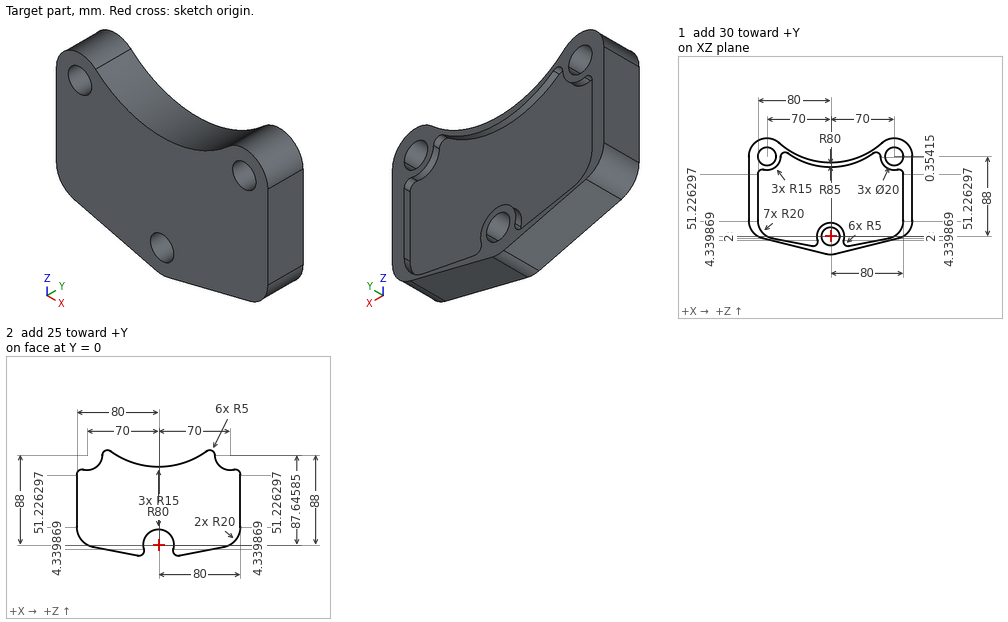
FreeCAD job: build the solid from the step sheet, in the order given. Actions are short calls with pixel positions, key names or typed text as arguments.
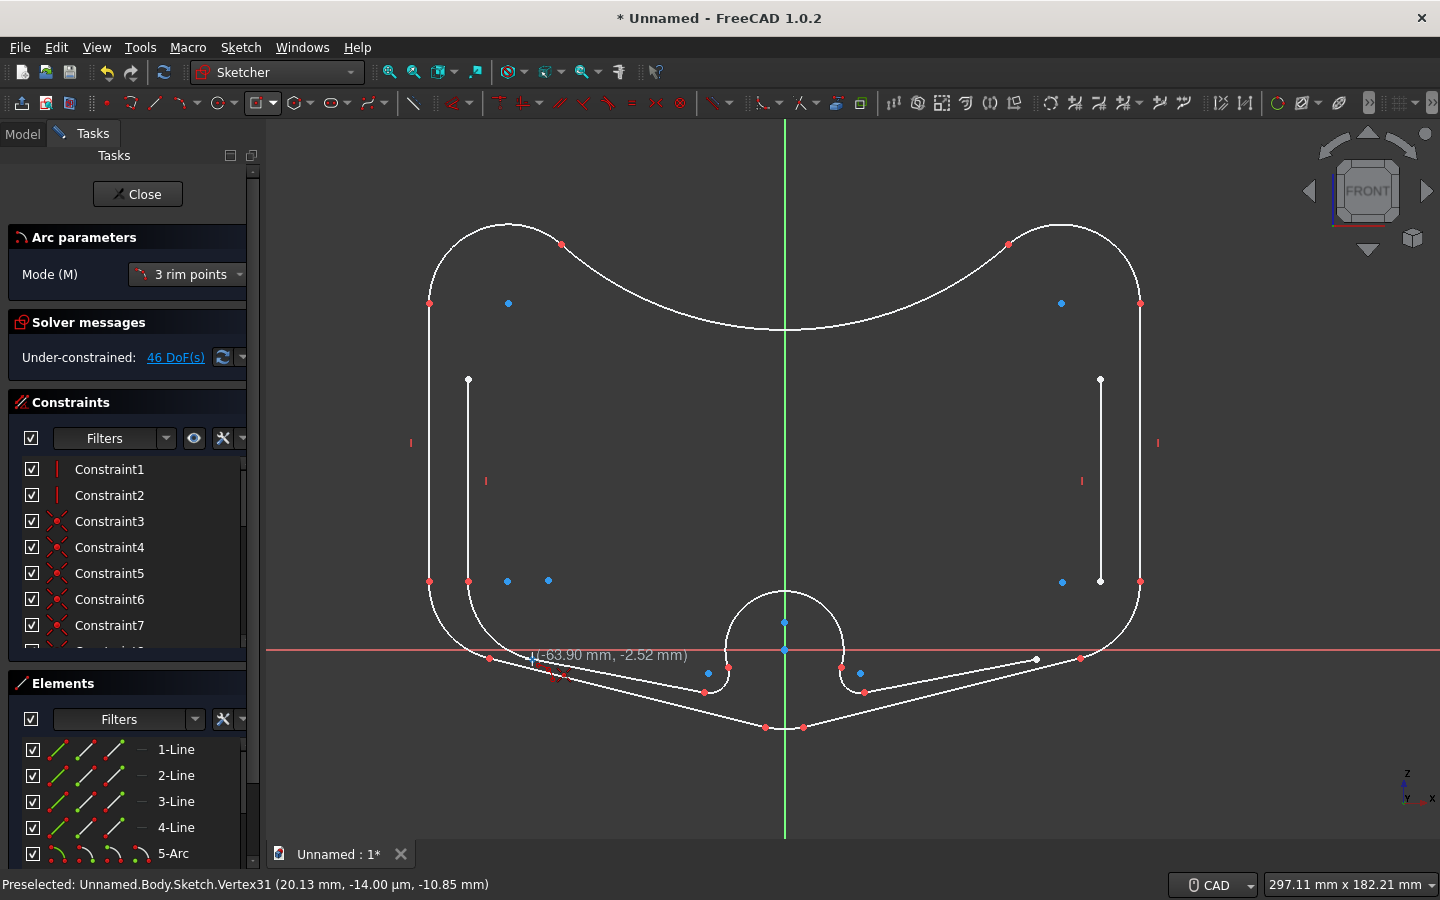
scroll(1037, 659, up, 3)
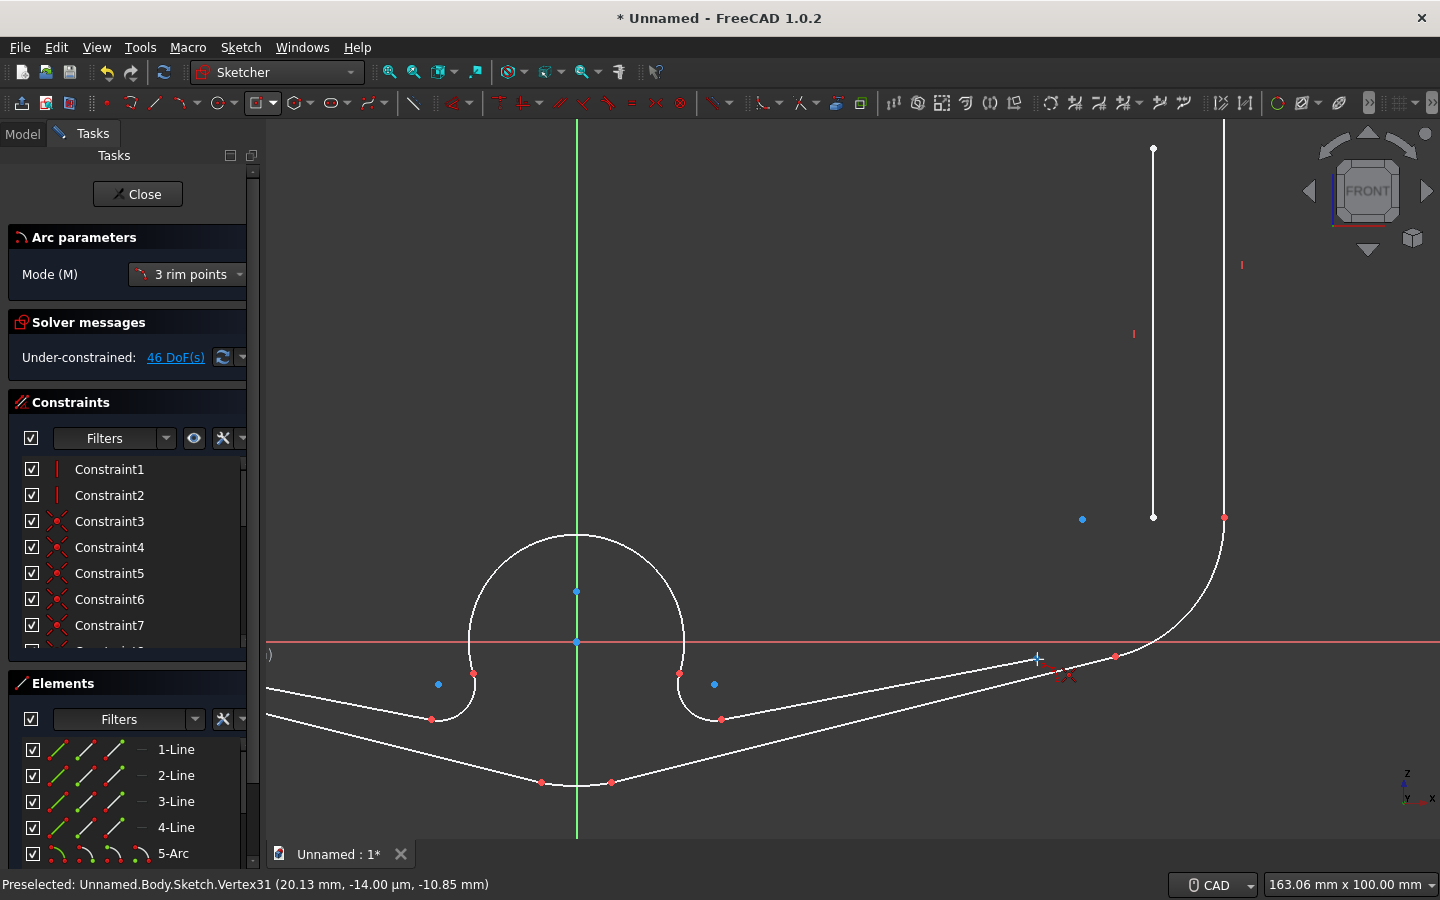
click(1036, 659)
click(1153, 518)
click(1120, 608)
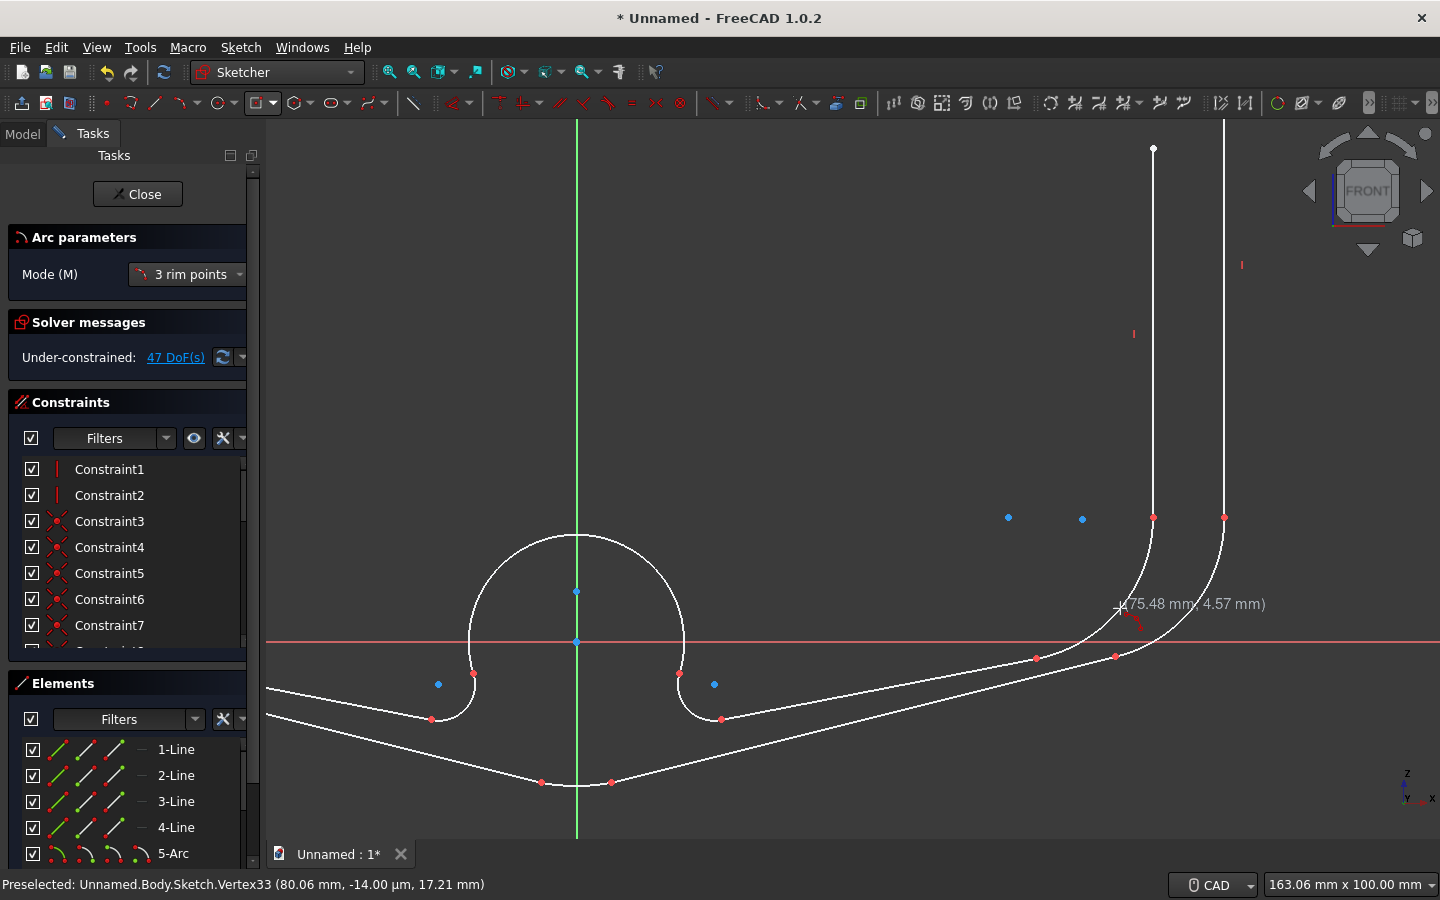
click(1153, 149)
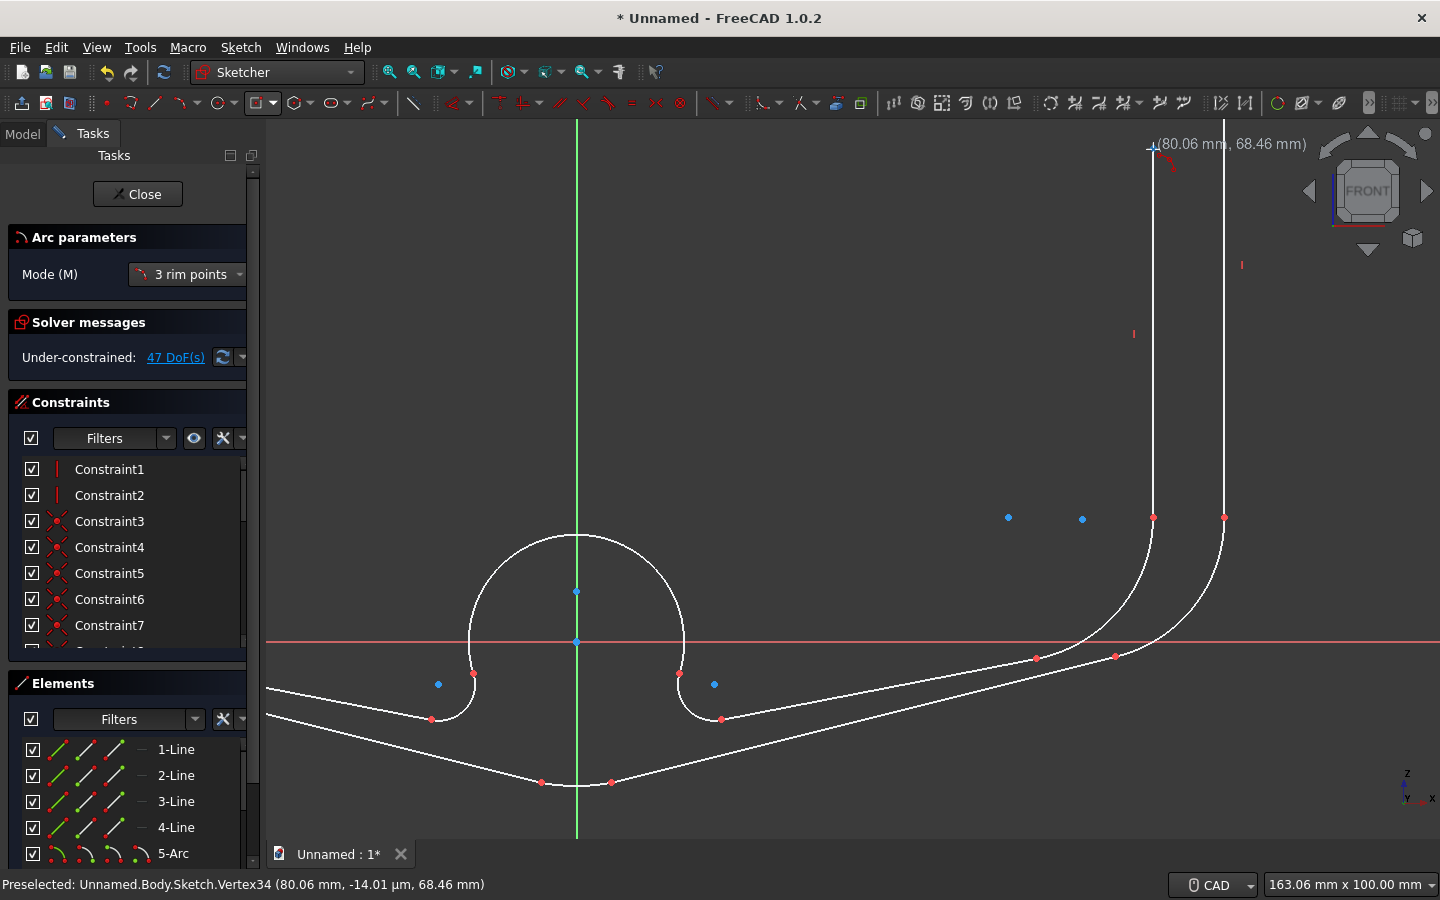
scroll(1037, 659, down, 3)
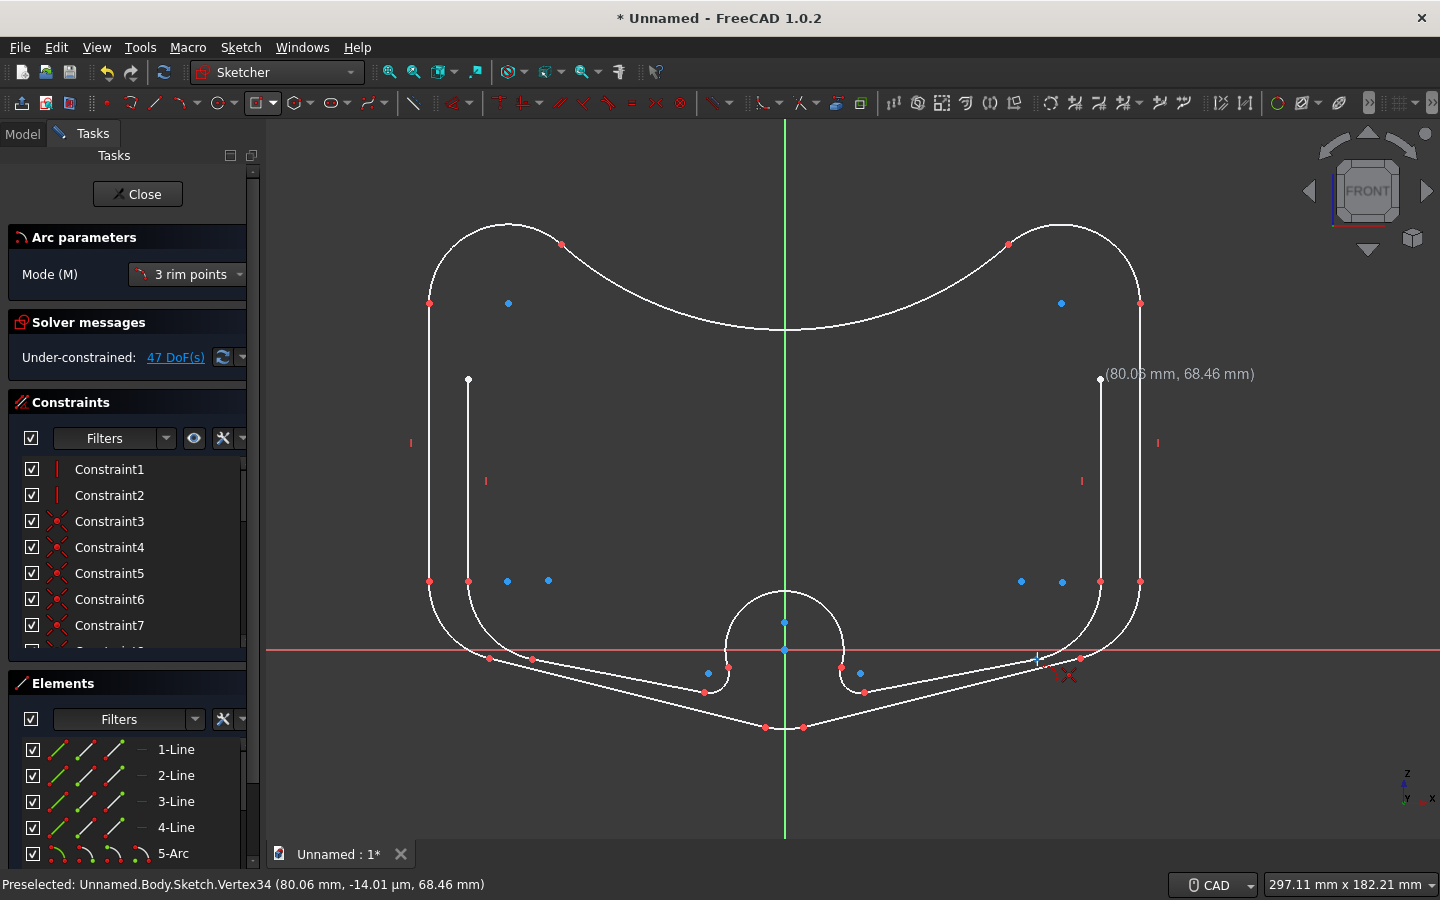
click(1076, 360)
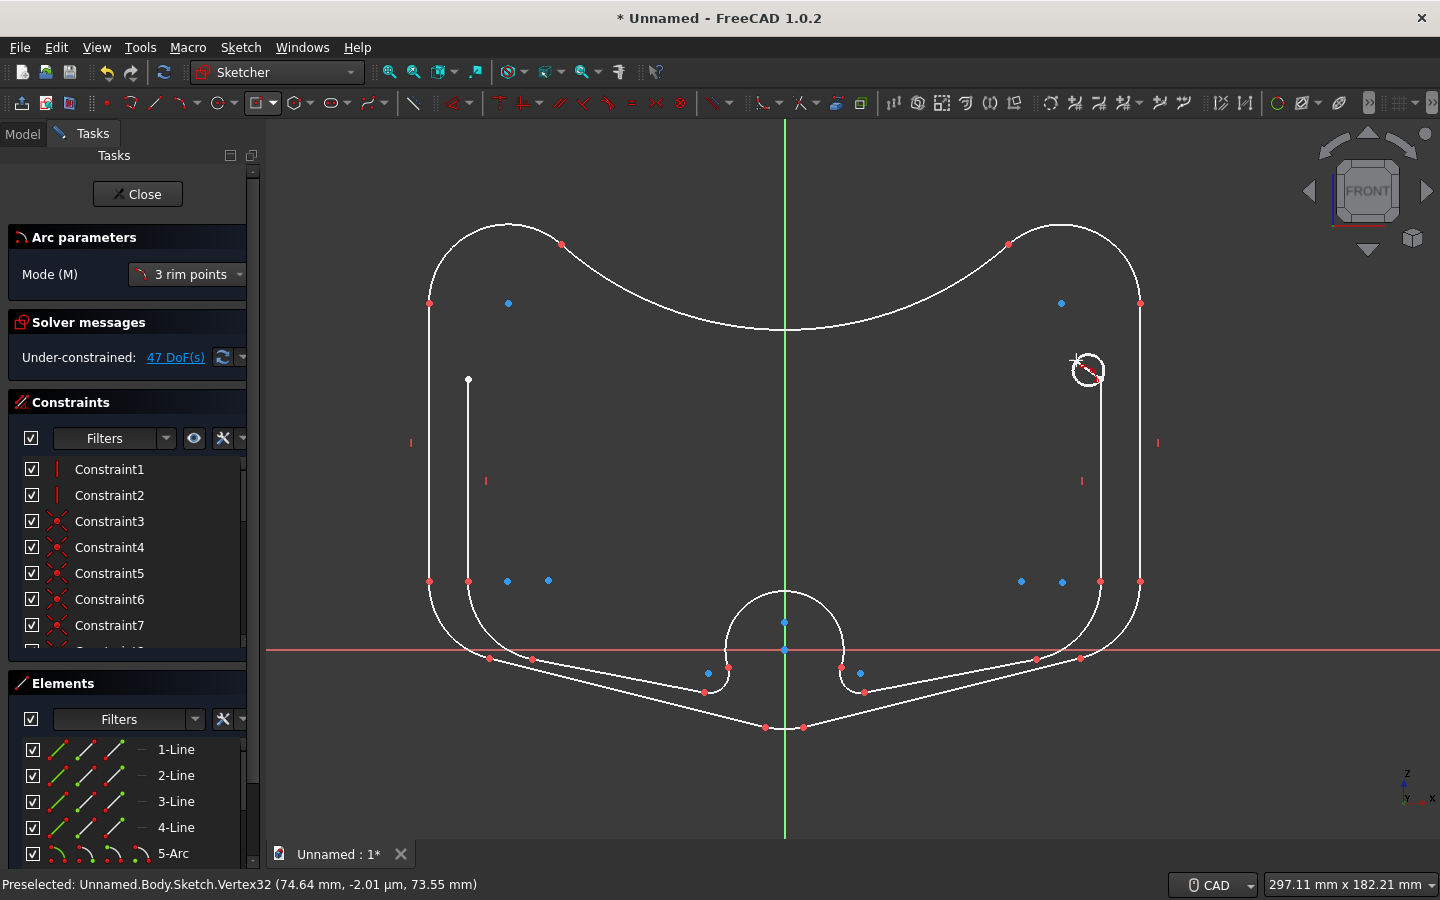
scroll(1093, 363, up, 4)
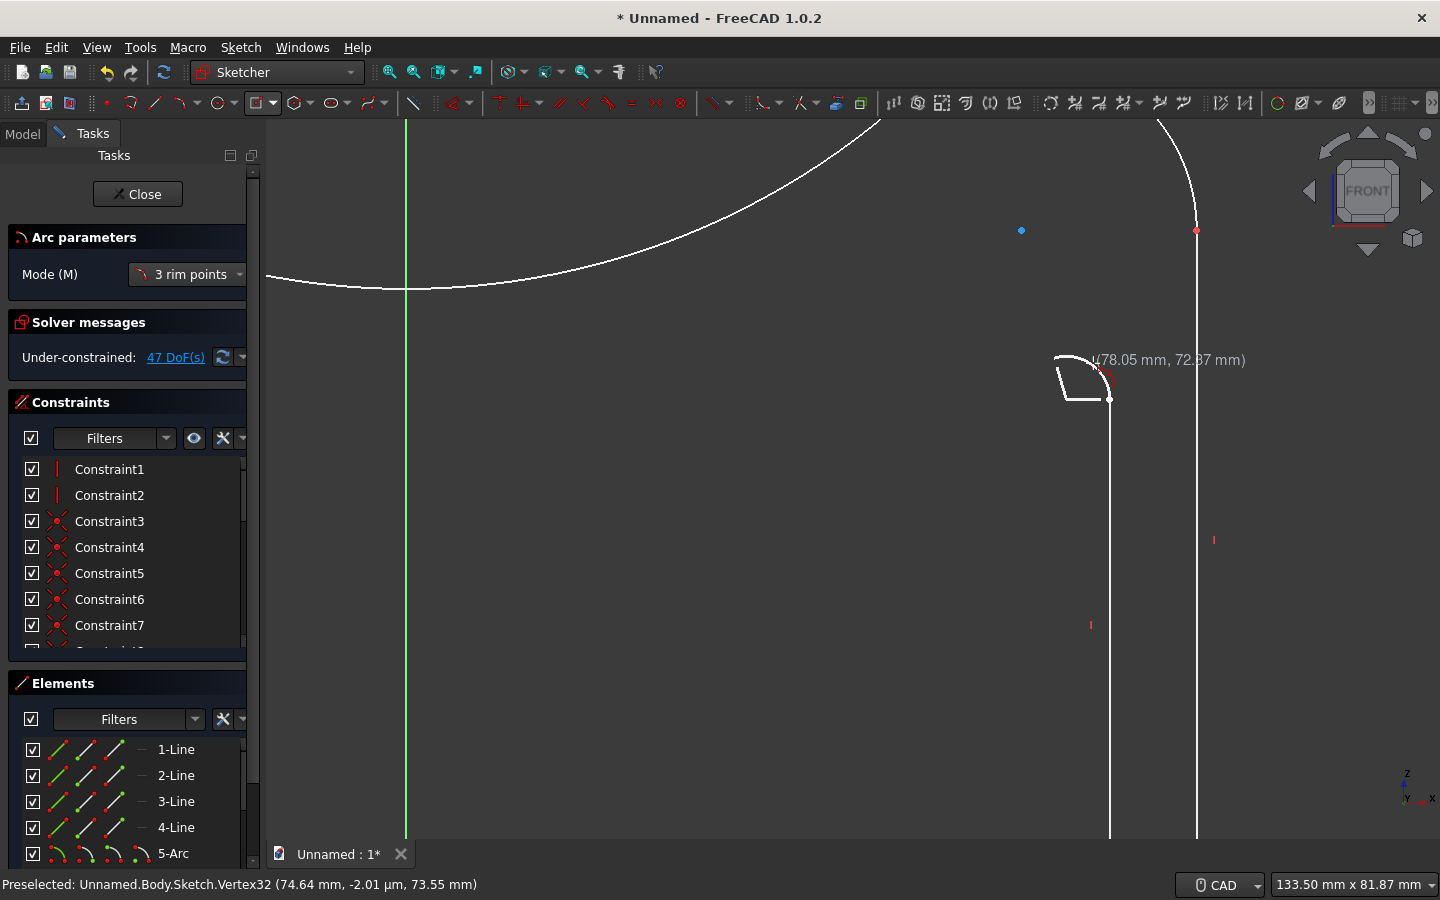
click(1092, 363)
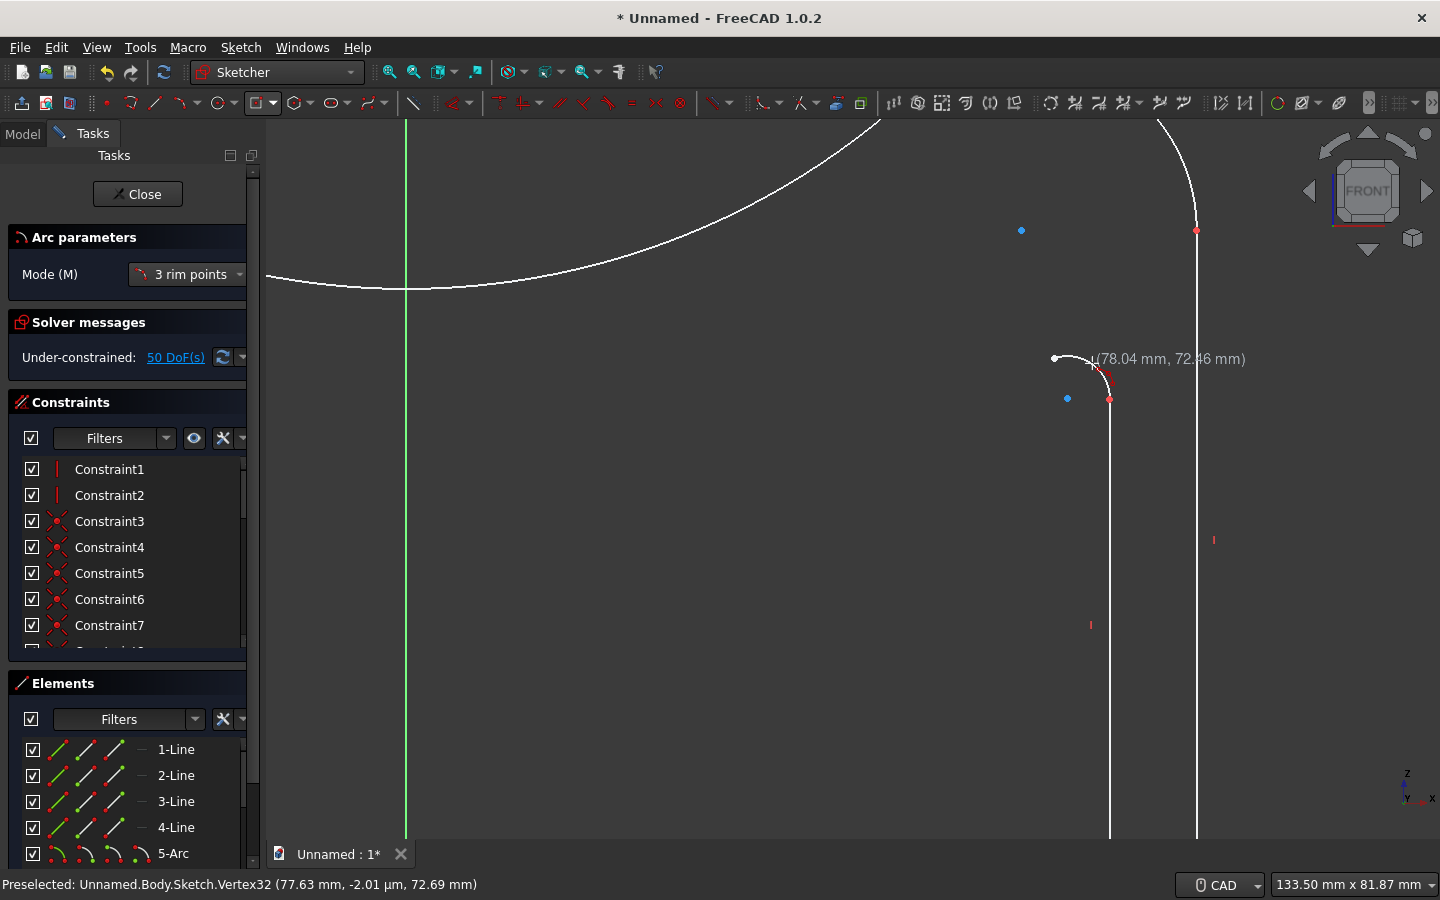
click(1054, 358)
click(889, 230)
click(942, 333)